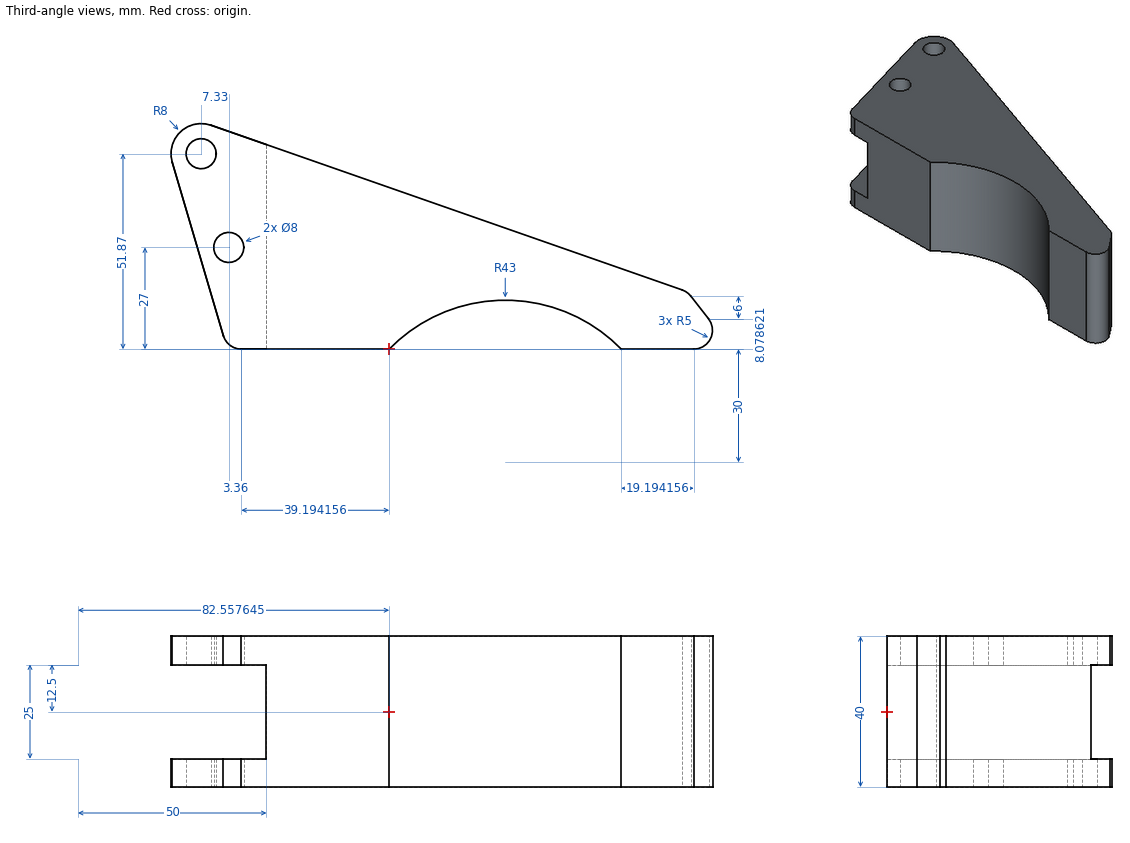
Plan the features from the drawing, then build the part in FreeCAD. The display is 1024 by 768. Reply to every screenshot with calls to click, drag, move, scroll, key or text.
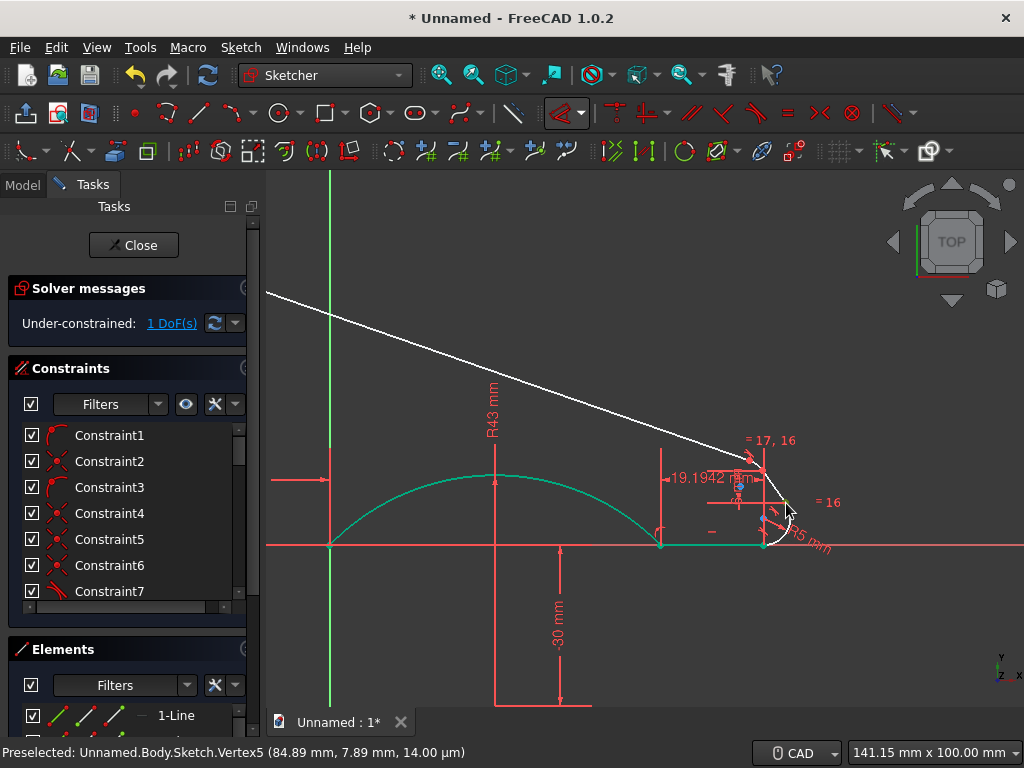
click(584, 114)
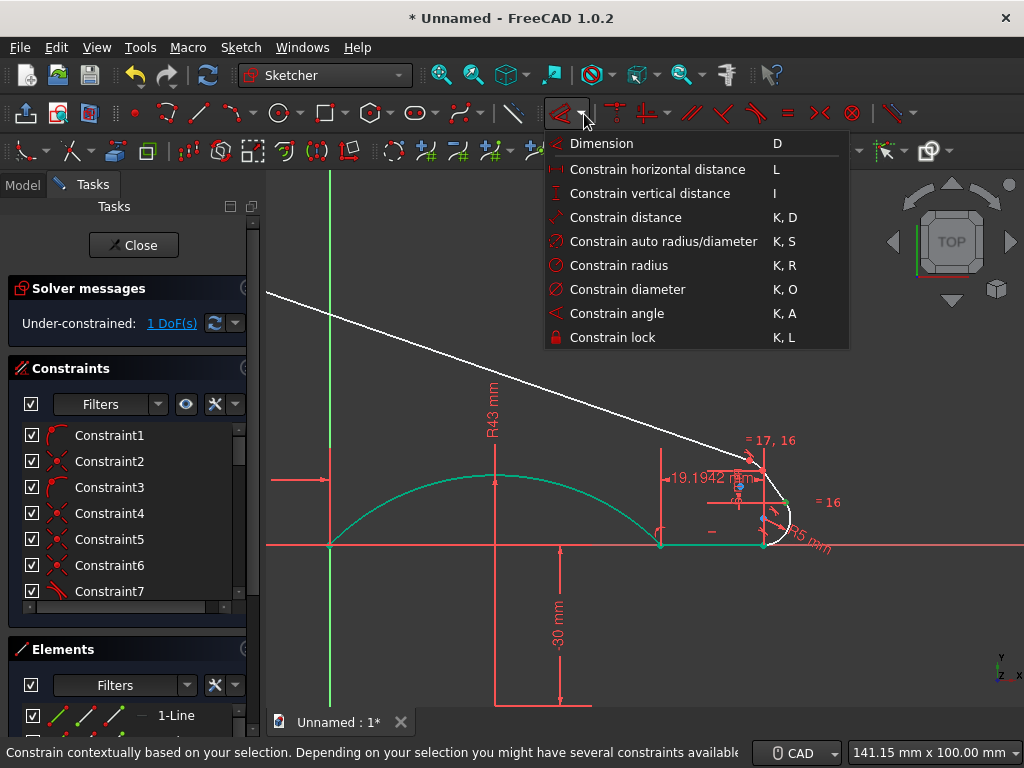
click(697, 193)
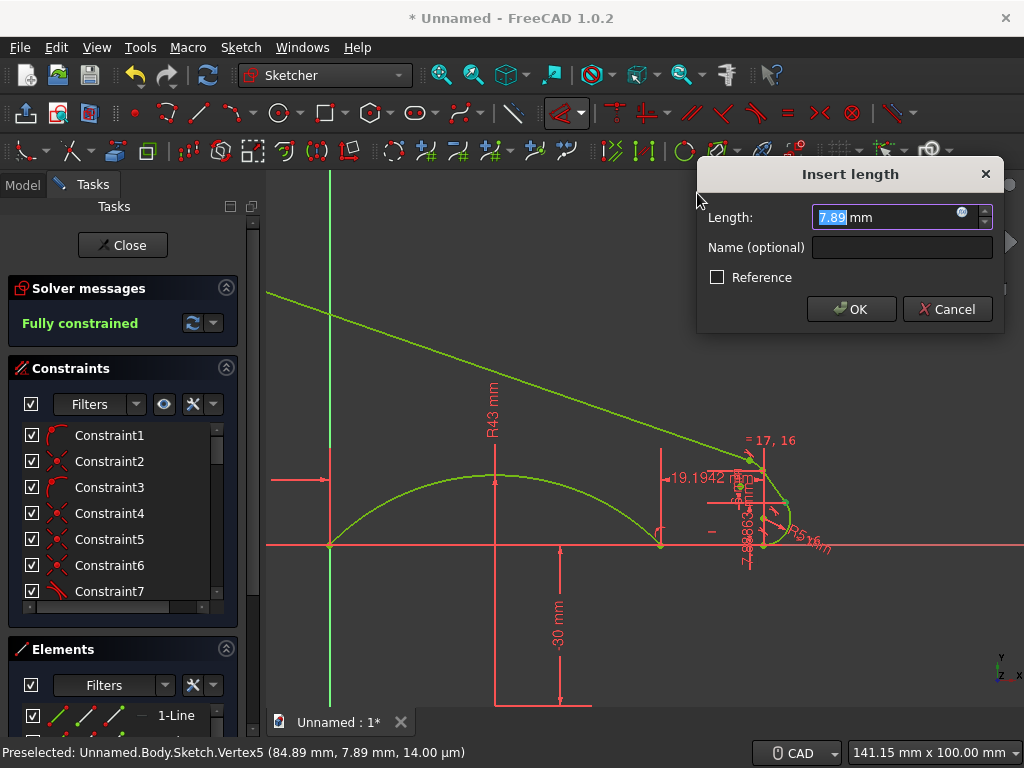
text(8.078621)
key(Return)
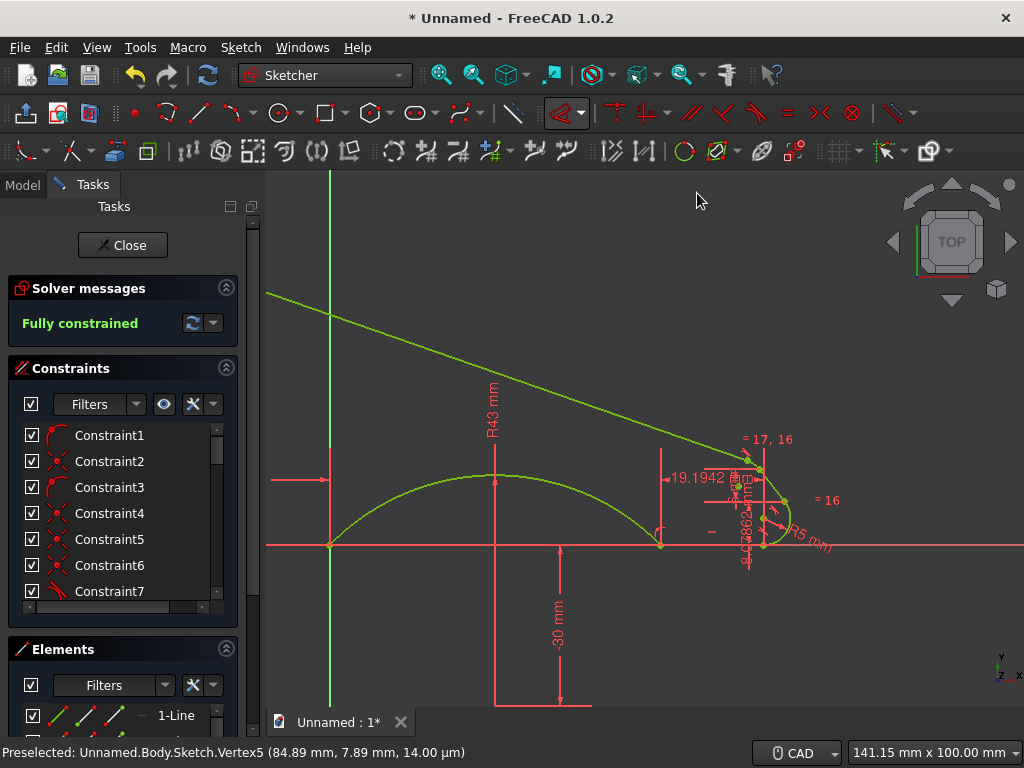
click(123, 245)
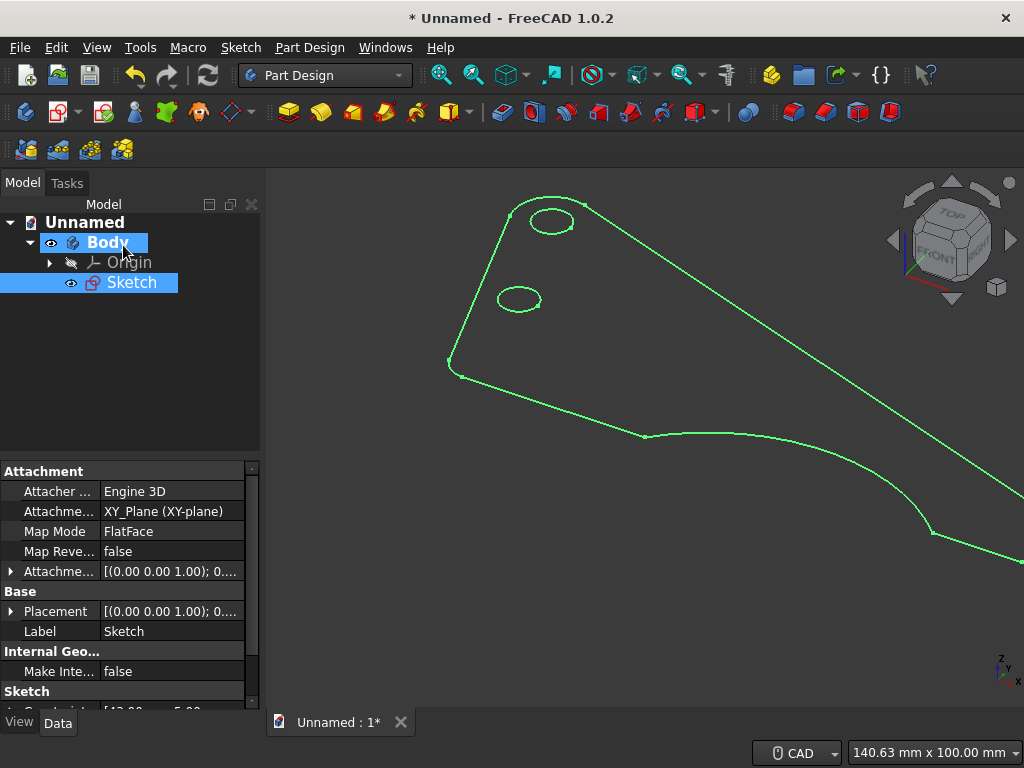
click(290, 112)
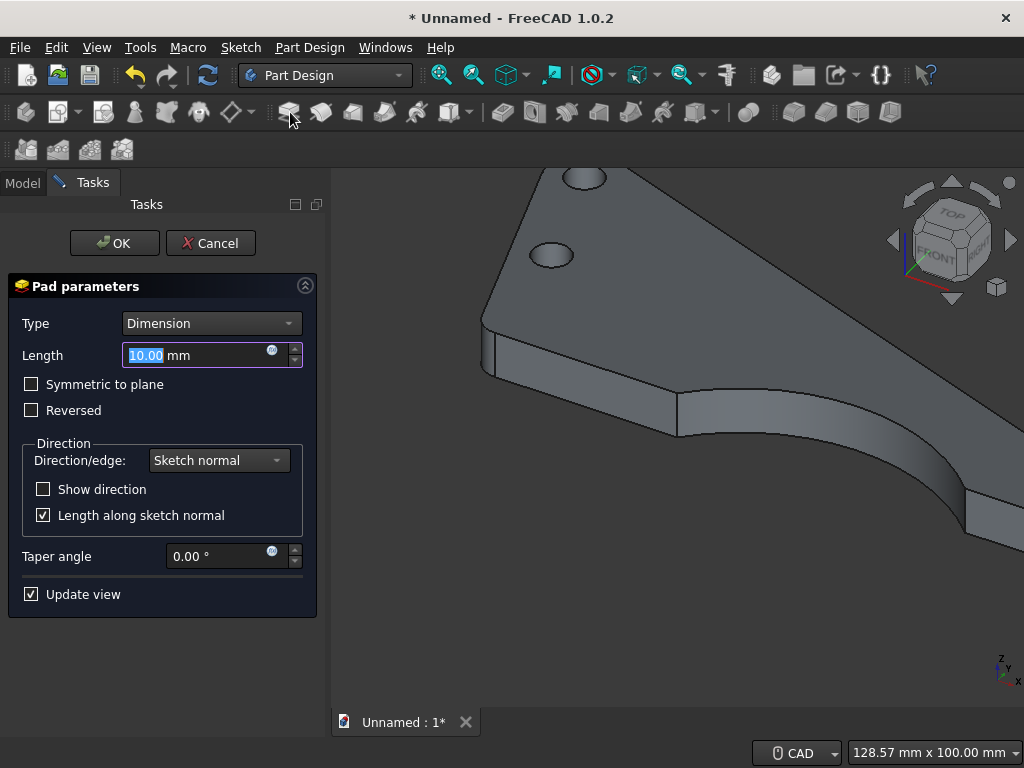
text(40)
key(Tab)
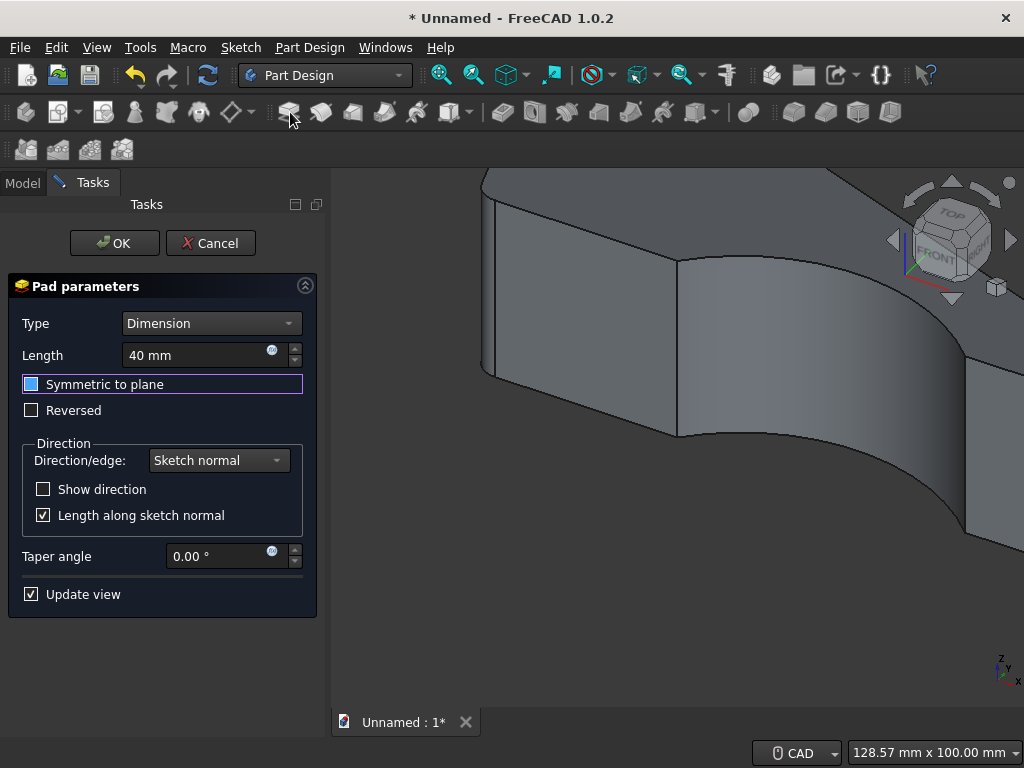
click(30, 384)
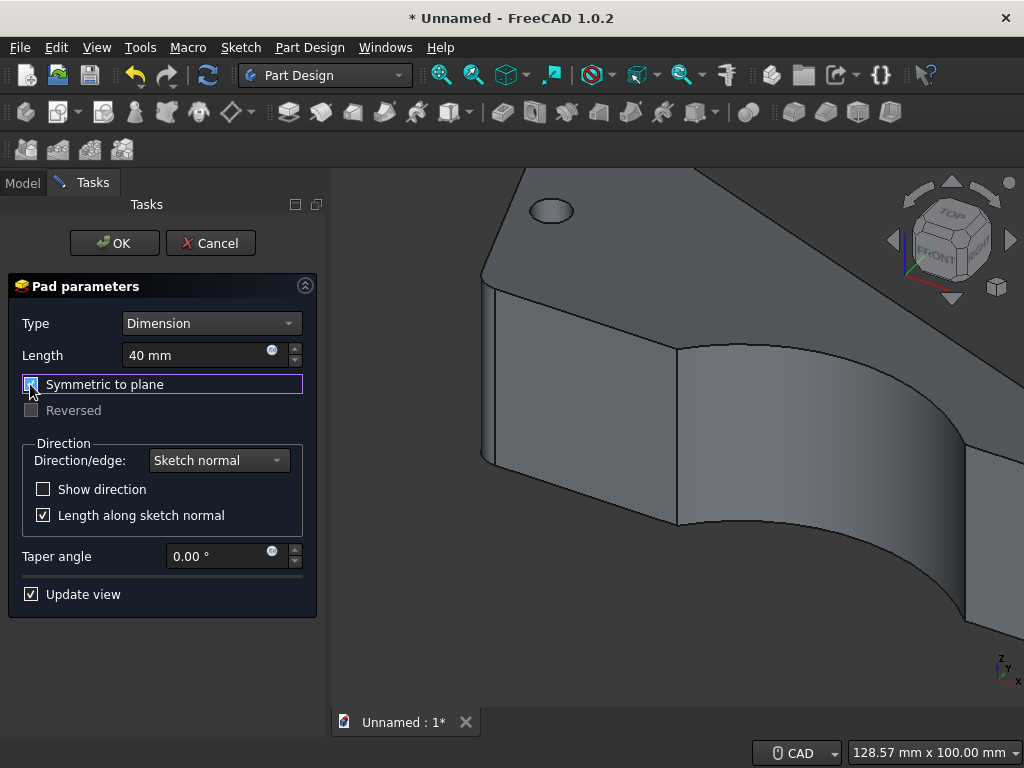
click(115, 243)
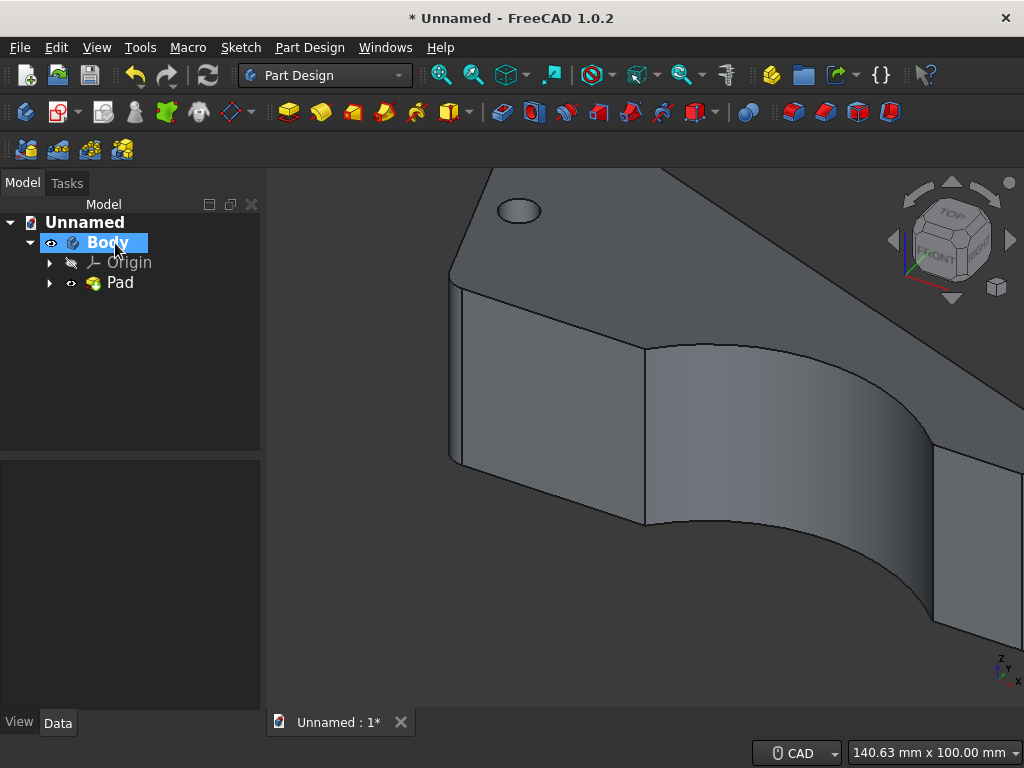
click(442, 76)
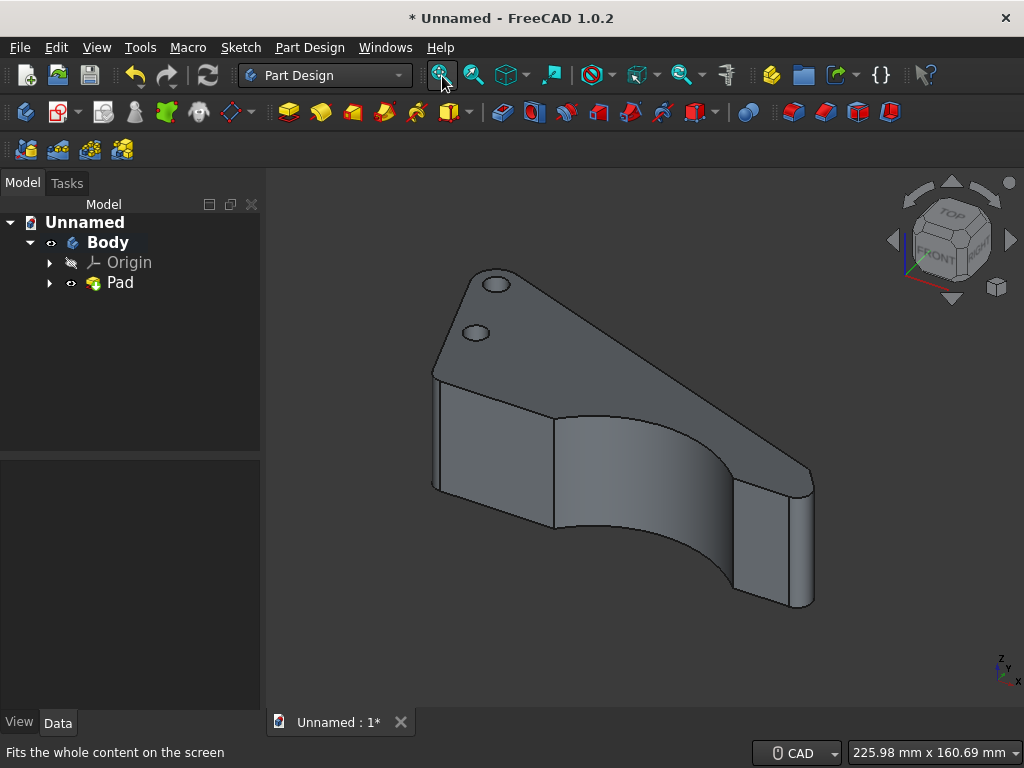
click(497, 454)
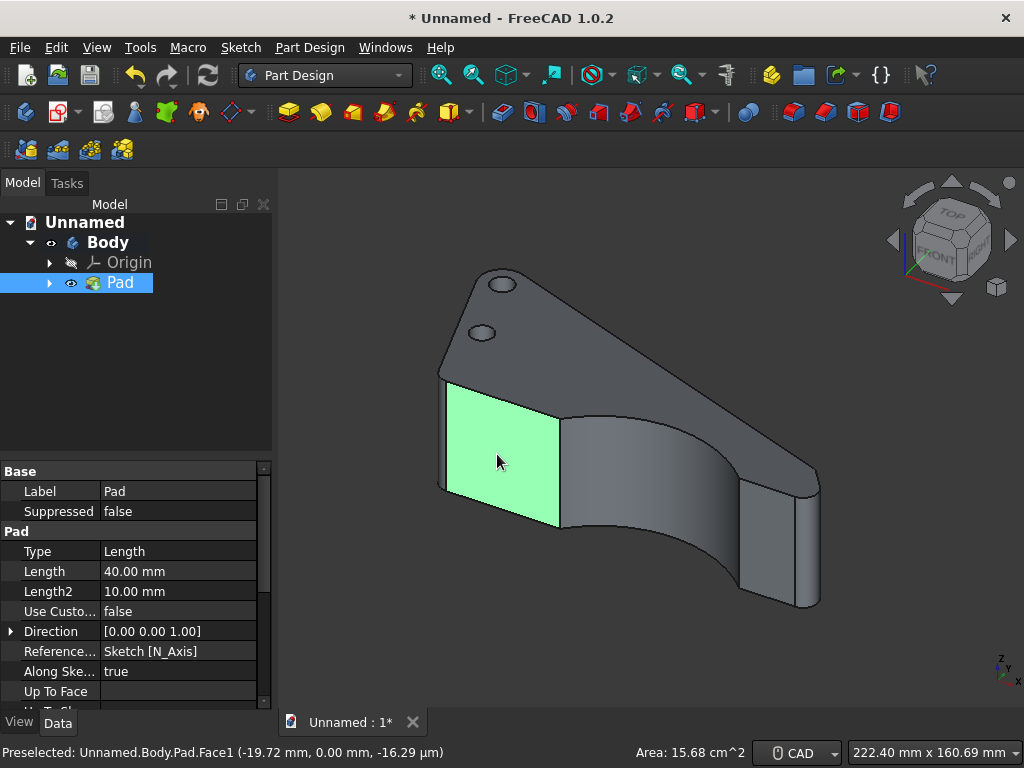
click(58, 112)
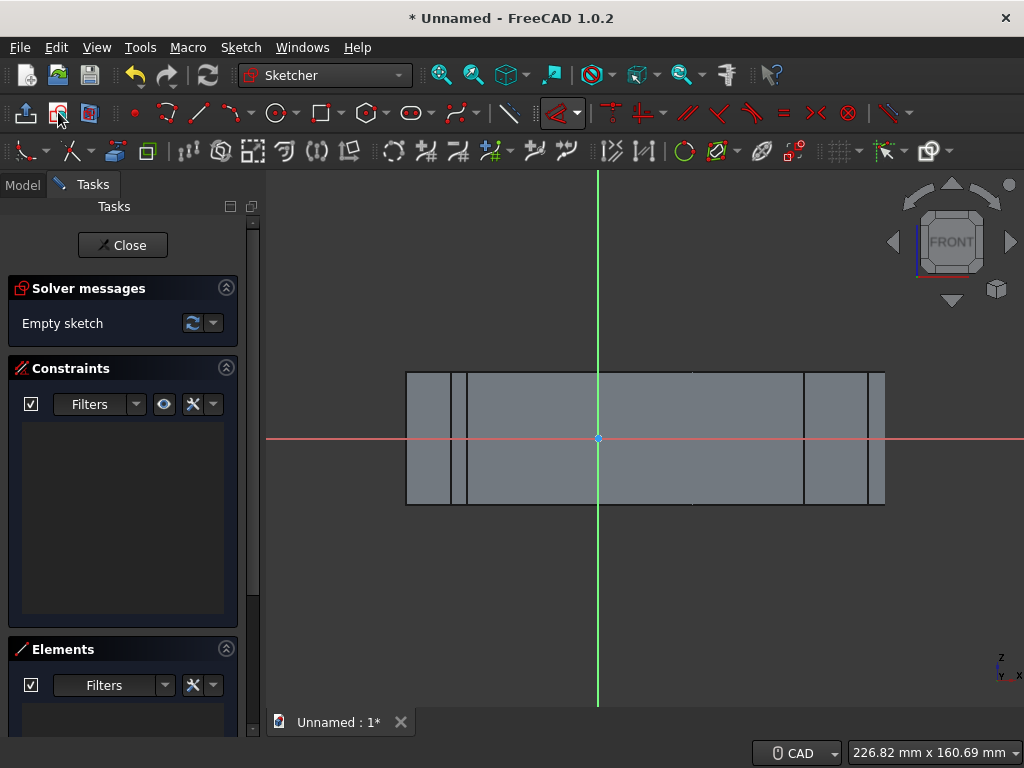
scroll(294, 439, up, 2)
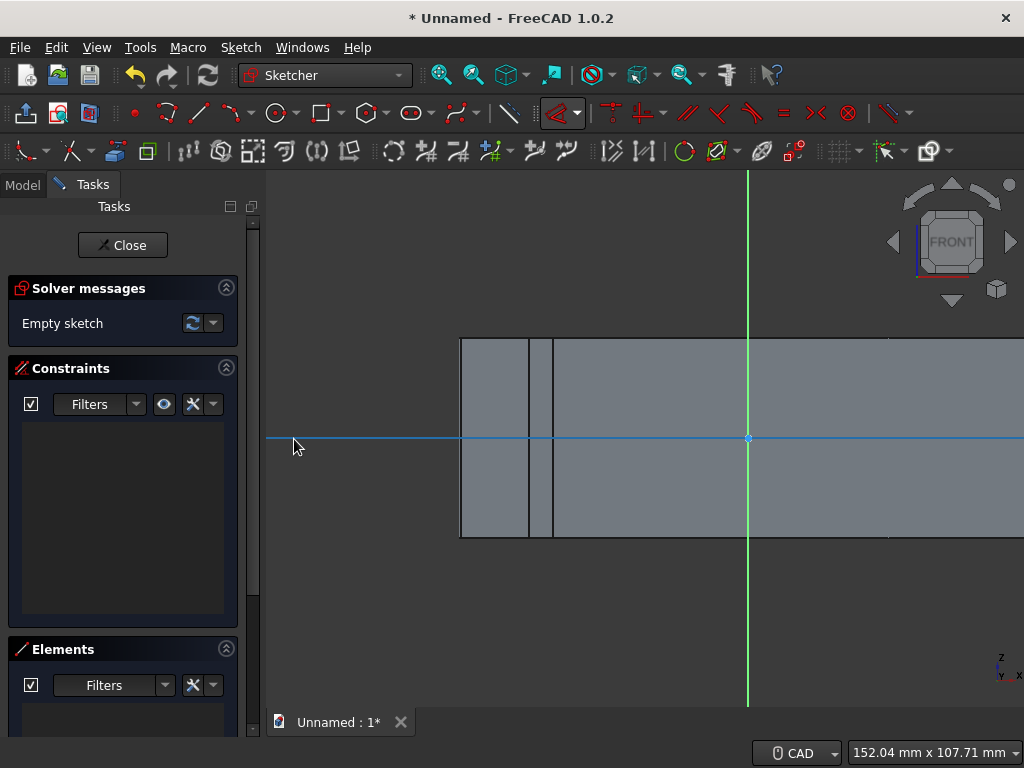
click(322, 114)